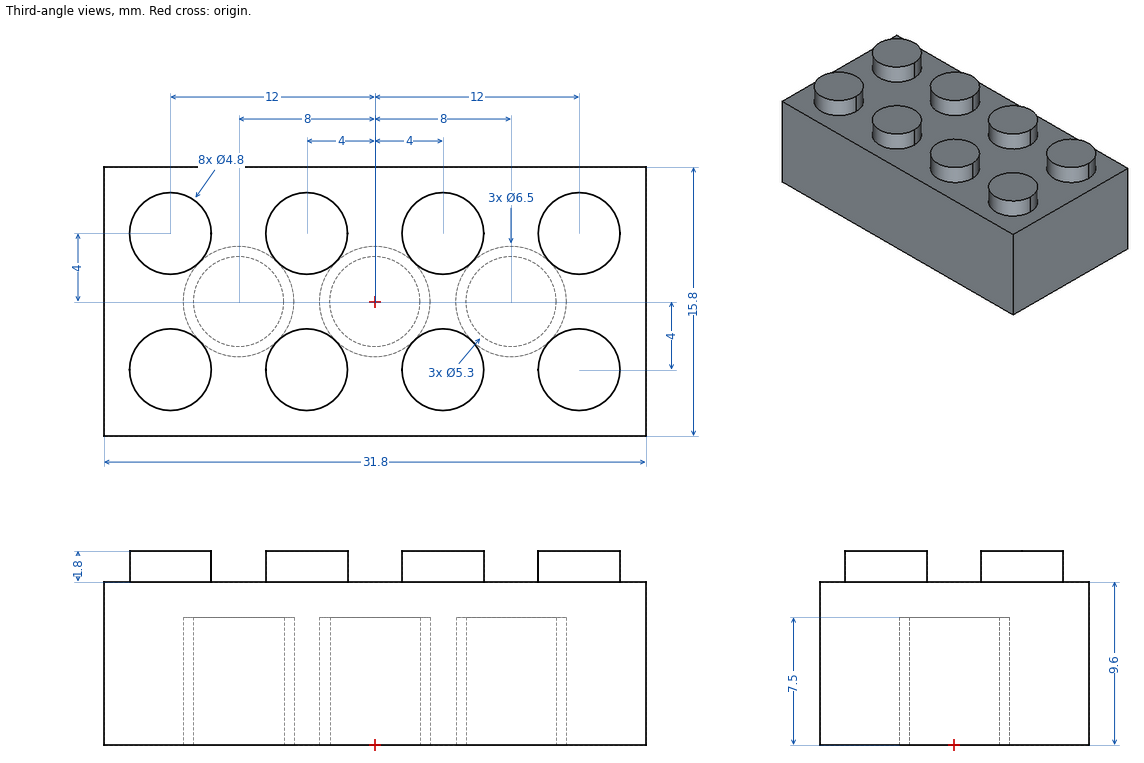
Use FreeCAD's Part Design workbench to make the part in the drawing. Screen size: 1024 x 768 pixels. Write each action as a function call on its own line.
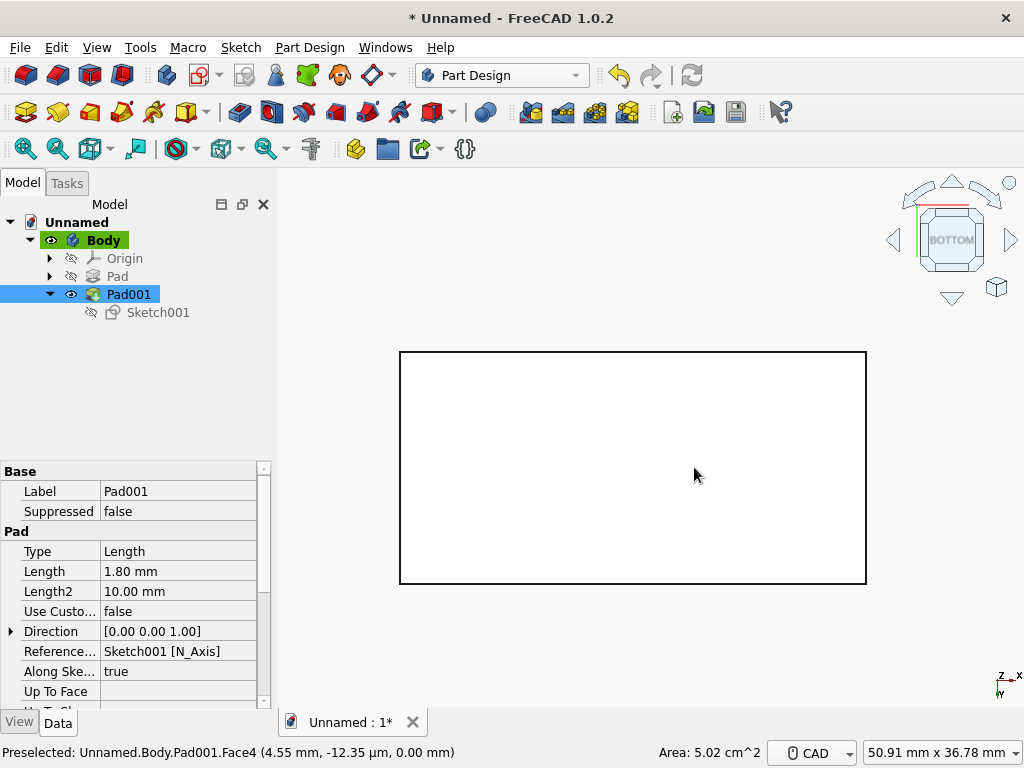
click(200, 76)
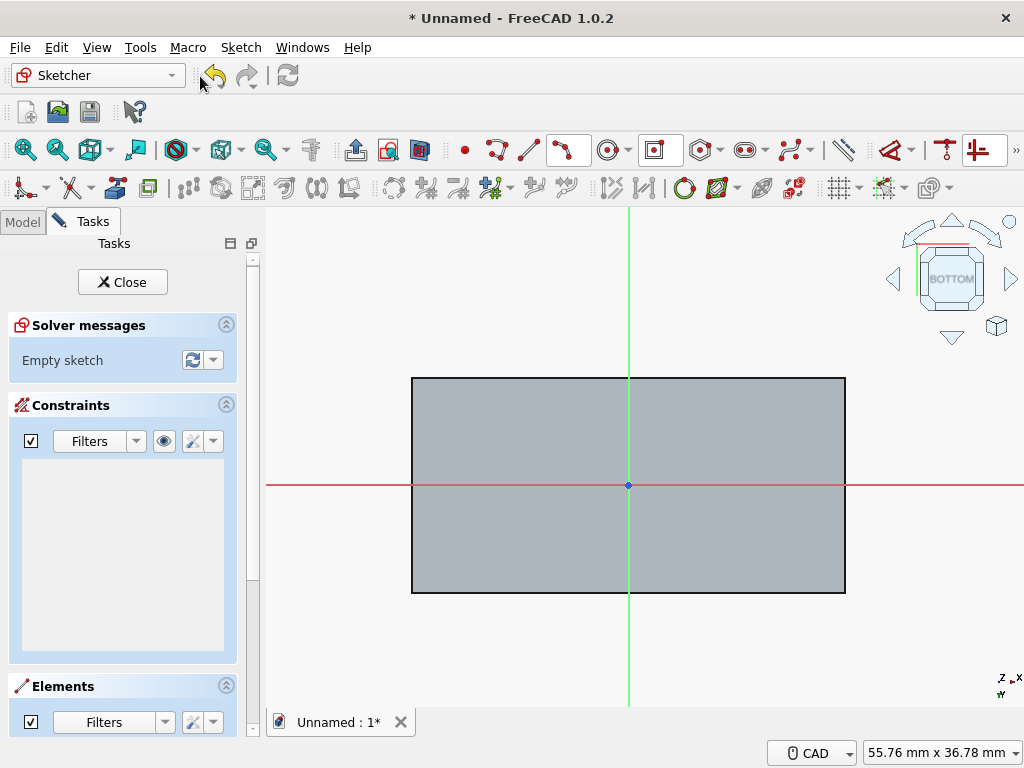
click(608, 150)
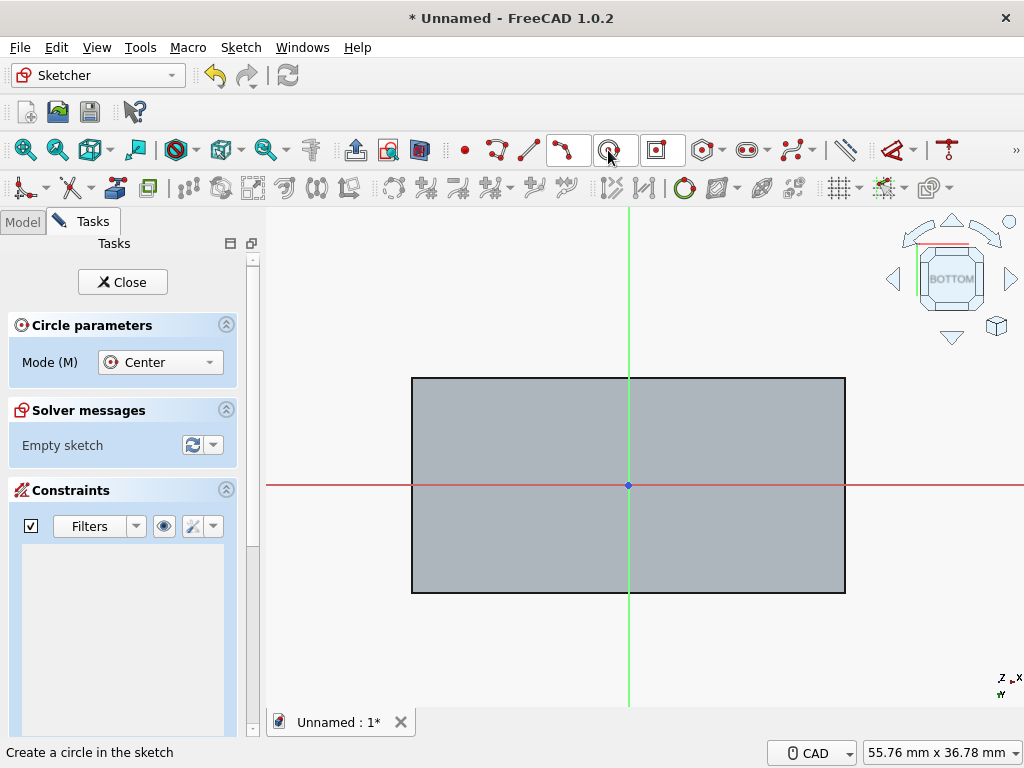
click(737, 485)
move(769, 454)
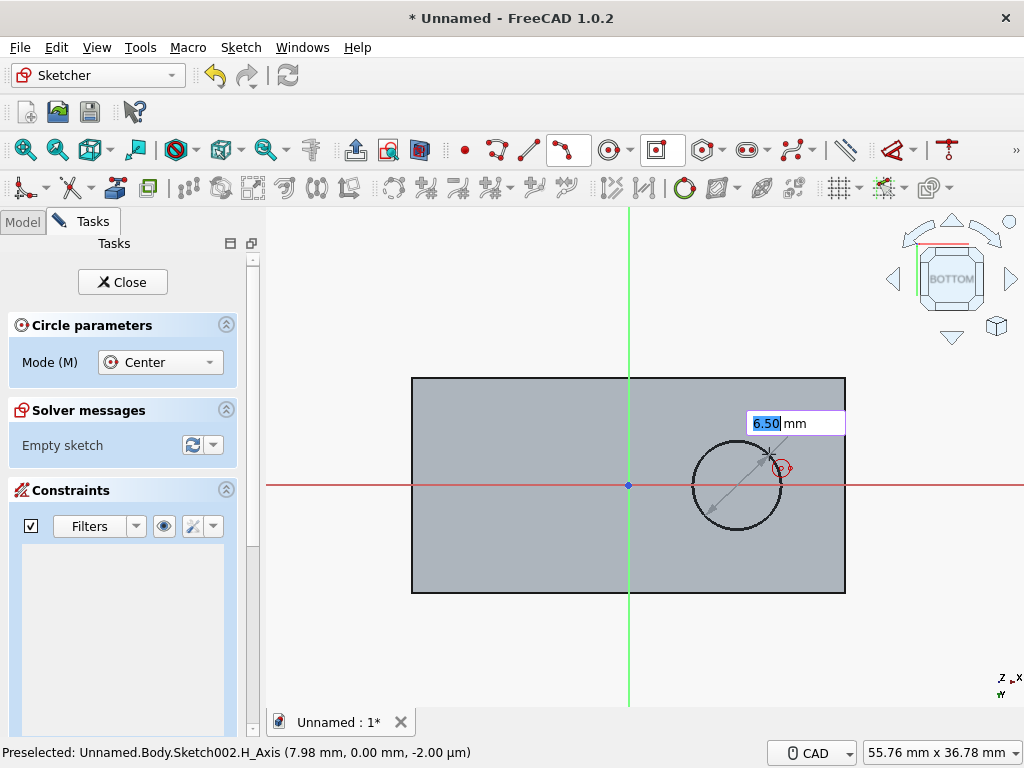
text(6.5)
key(Return)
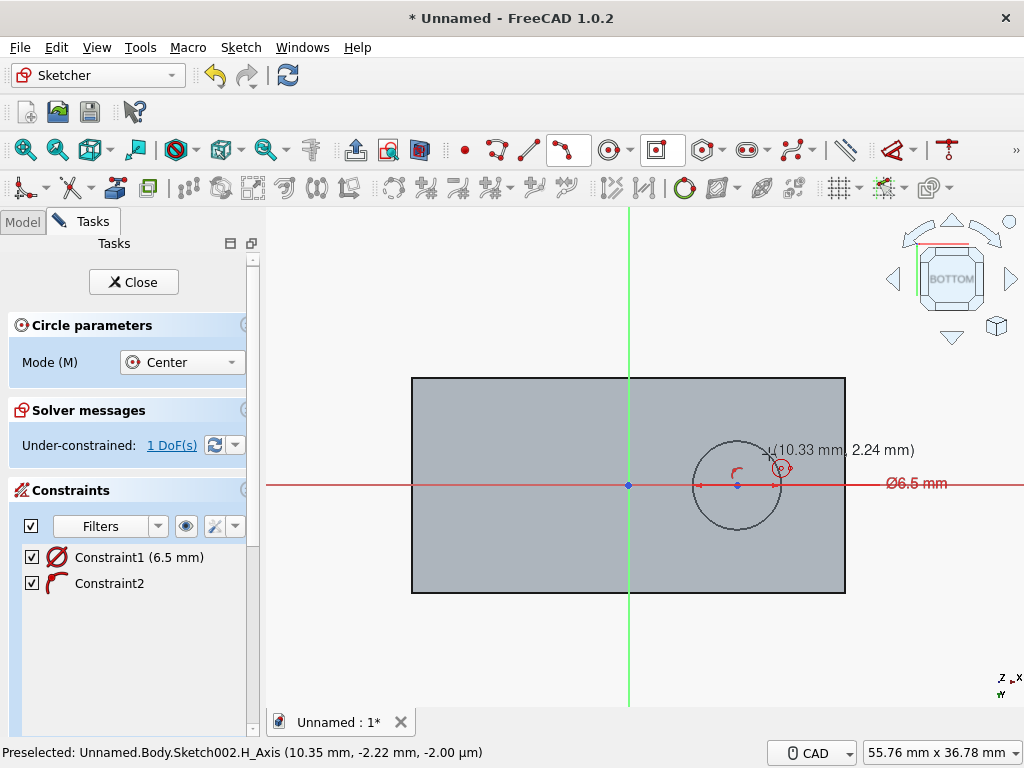
click(629, 485)
move(660, 454)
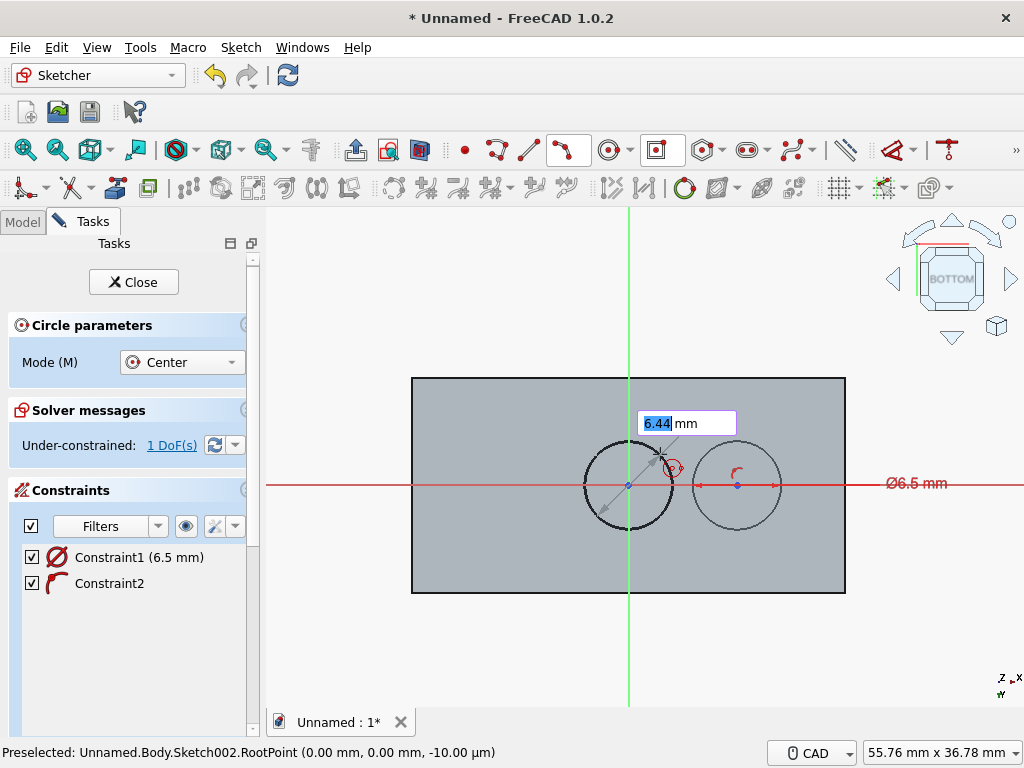
text(6.5)
key(Return)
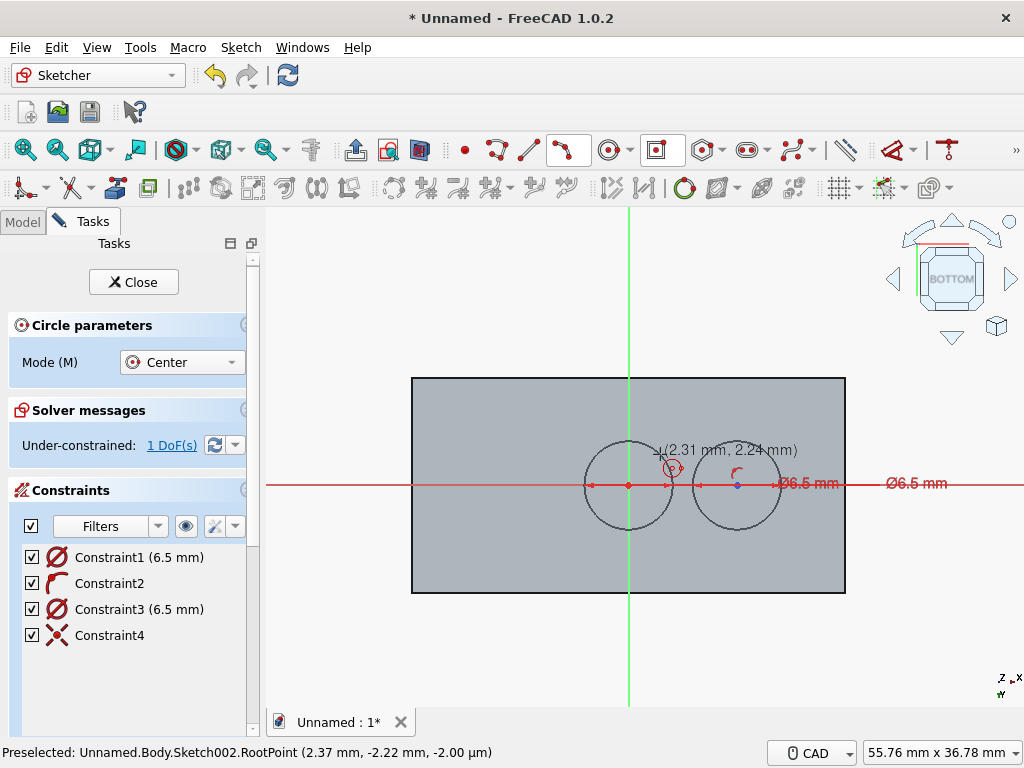
click(520, 485)
move(551, 454)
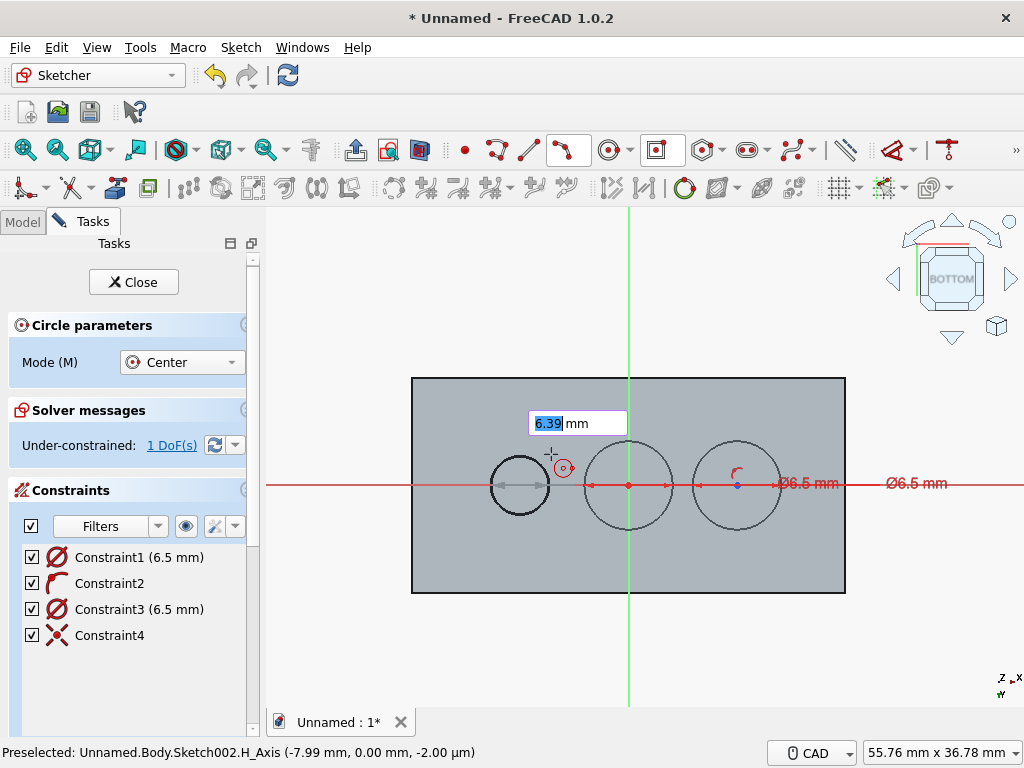
text(6.5)
key(Return)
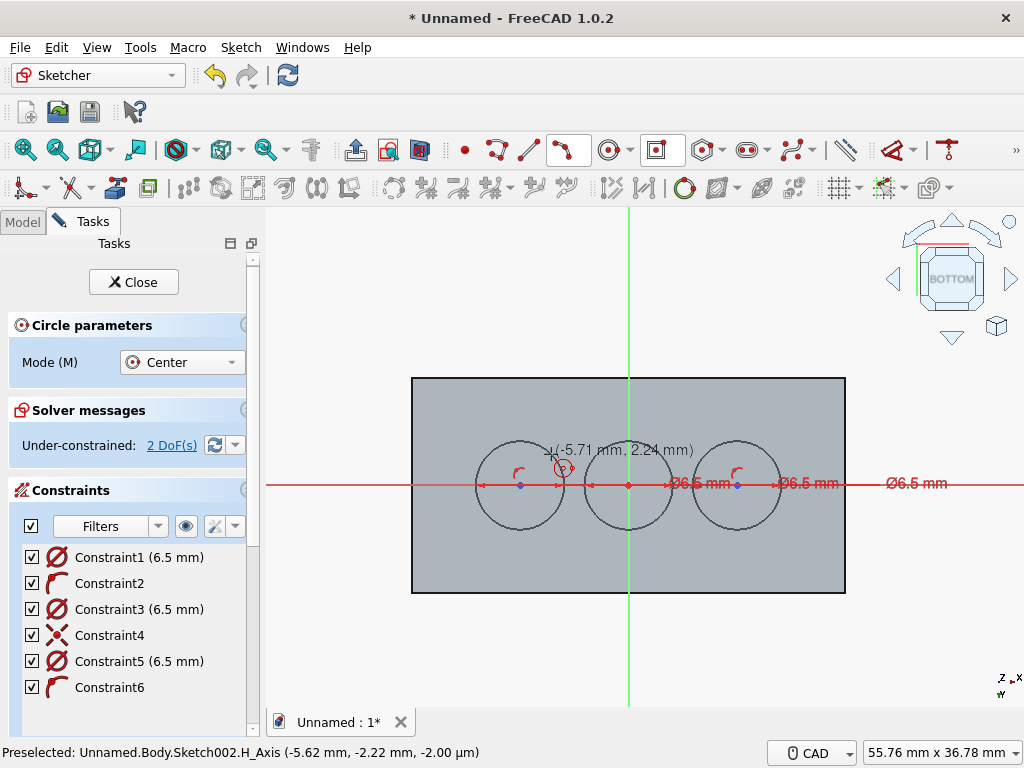
click(737, 485)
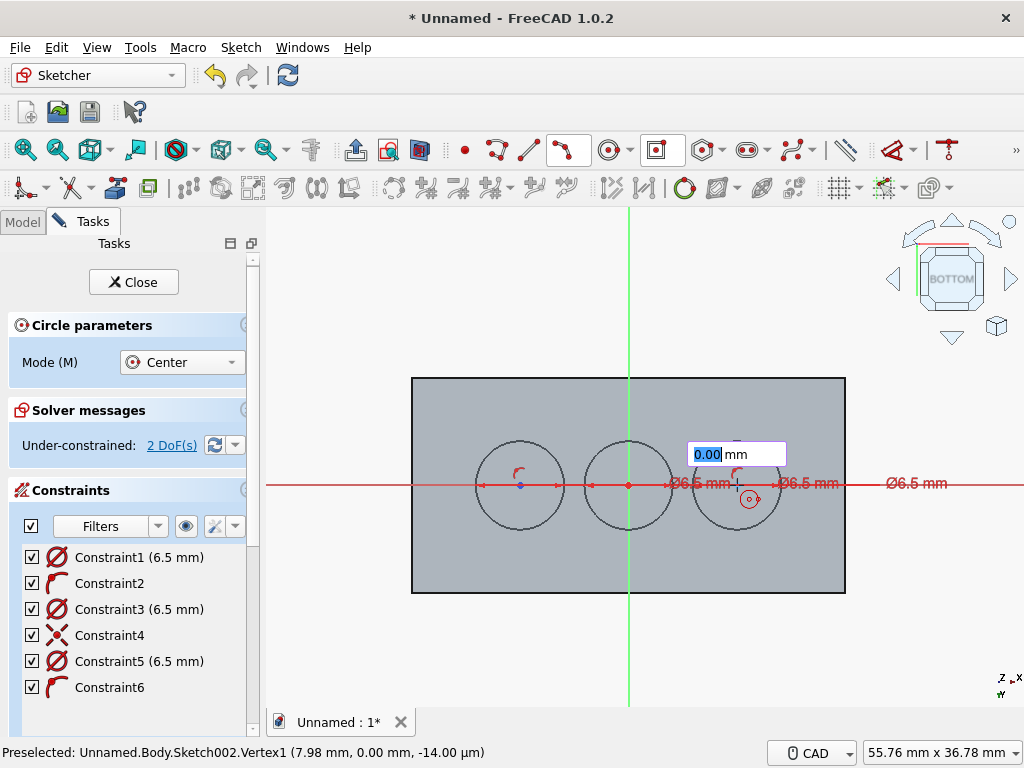
scroll(763, 460, up, 4)
move(762, 459)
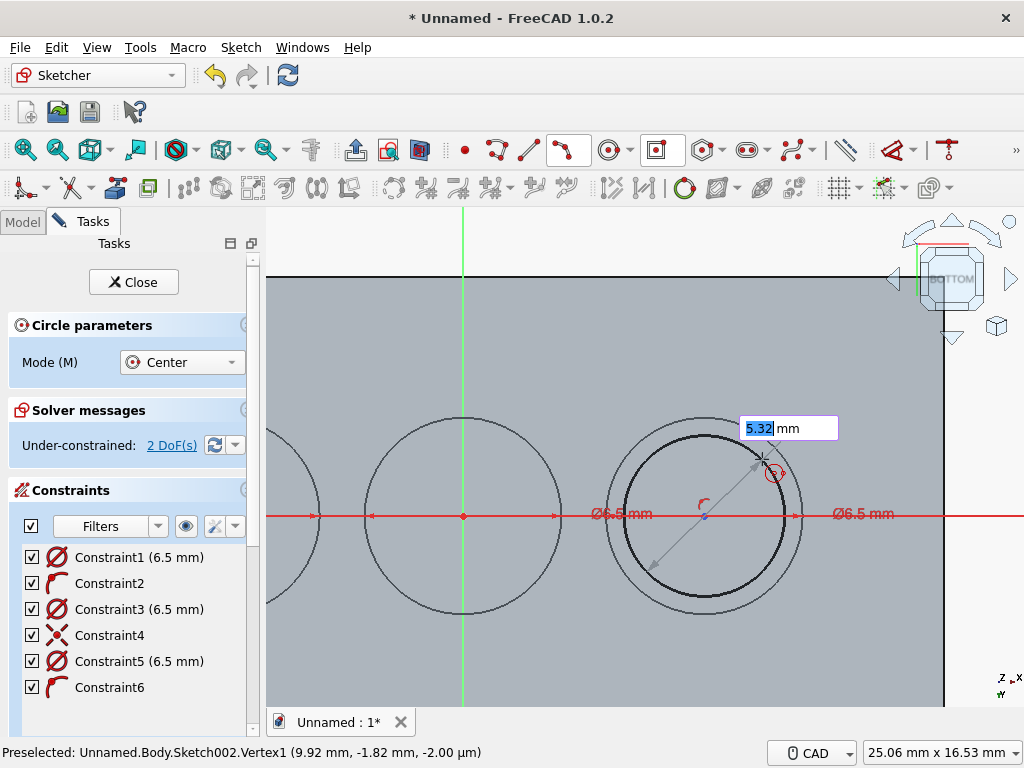
text(5.3)
key(Return)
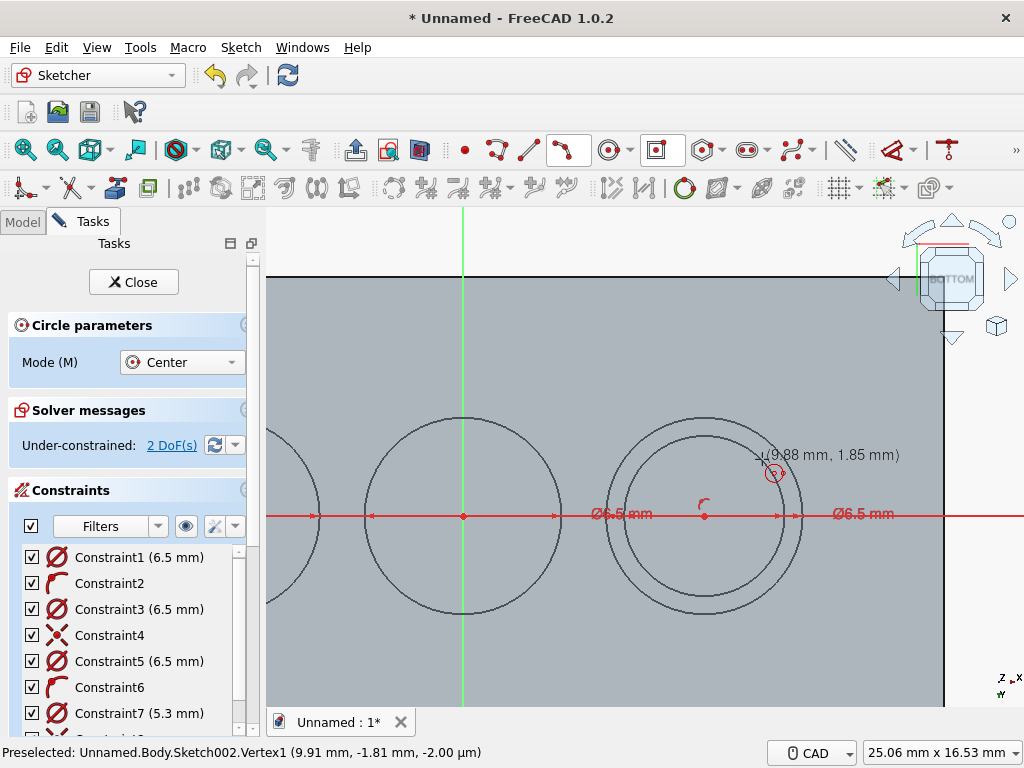
click(463, 516)
move(520, 459)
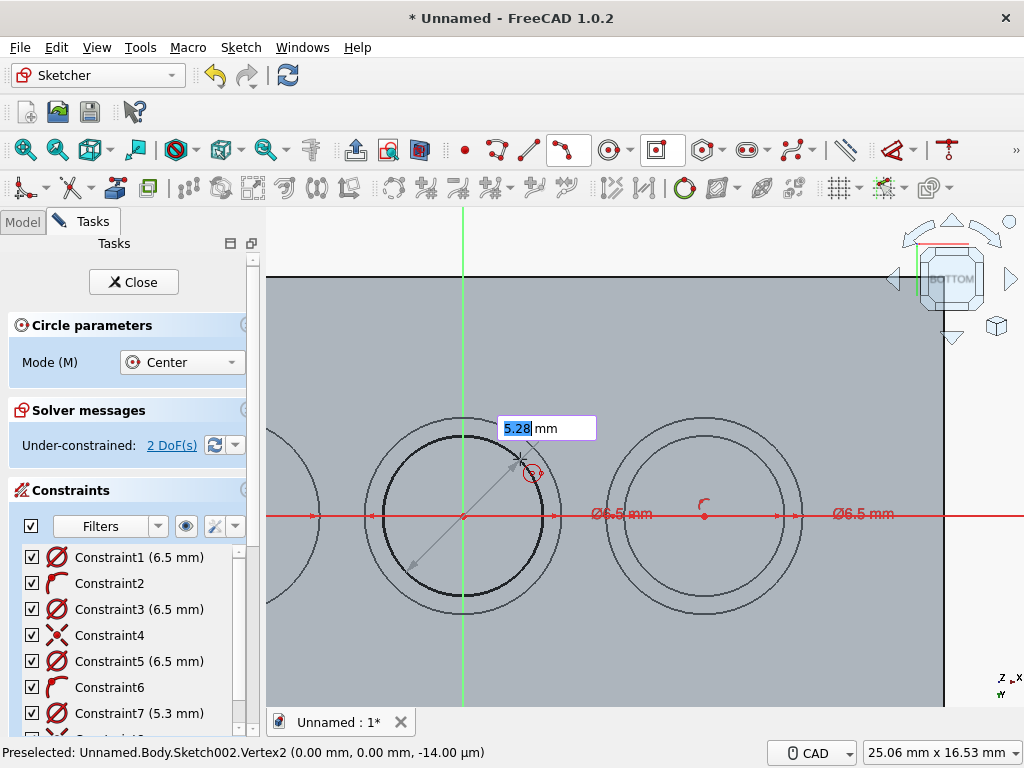
text(5.3)
key(Return)